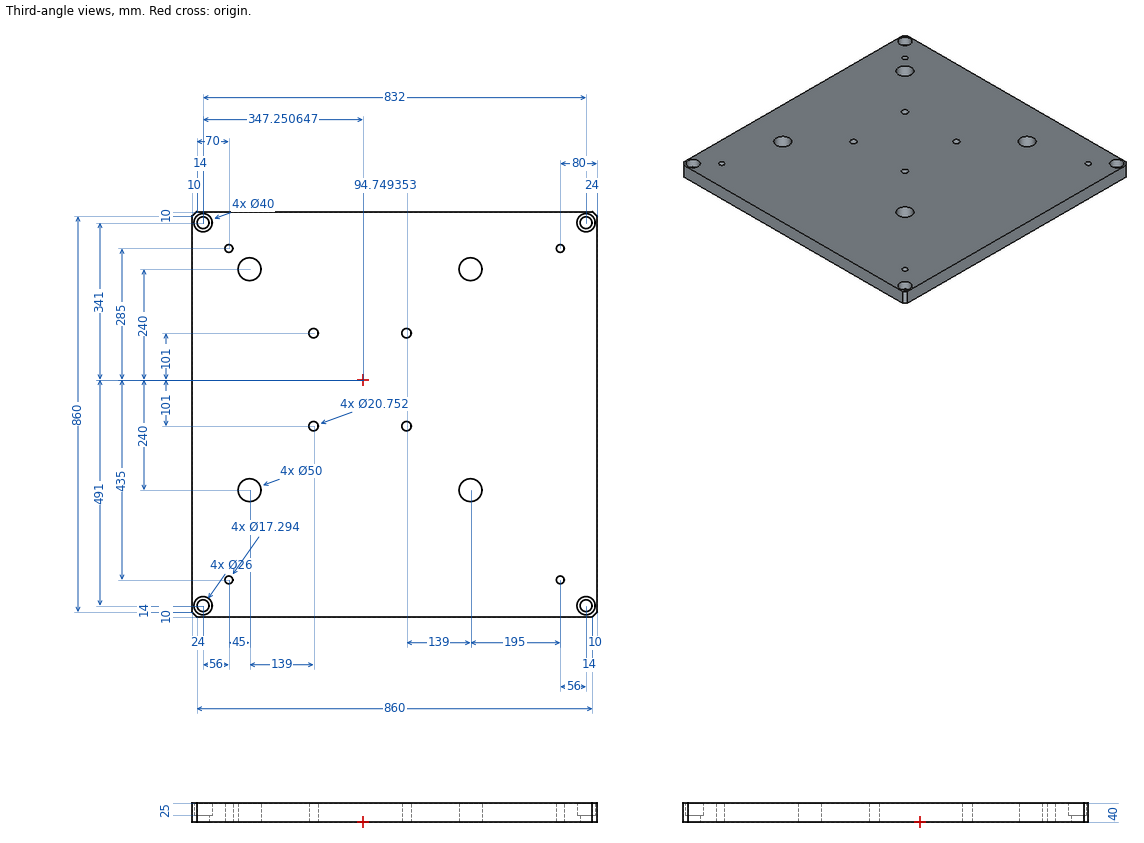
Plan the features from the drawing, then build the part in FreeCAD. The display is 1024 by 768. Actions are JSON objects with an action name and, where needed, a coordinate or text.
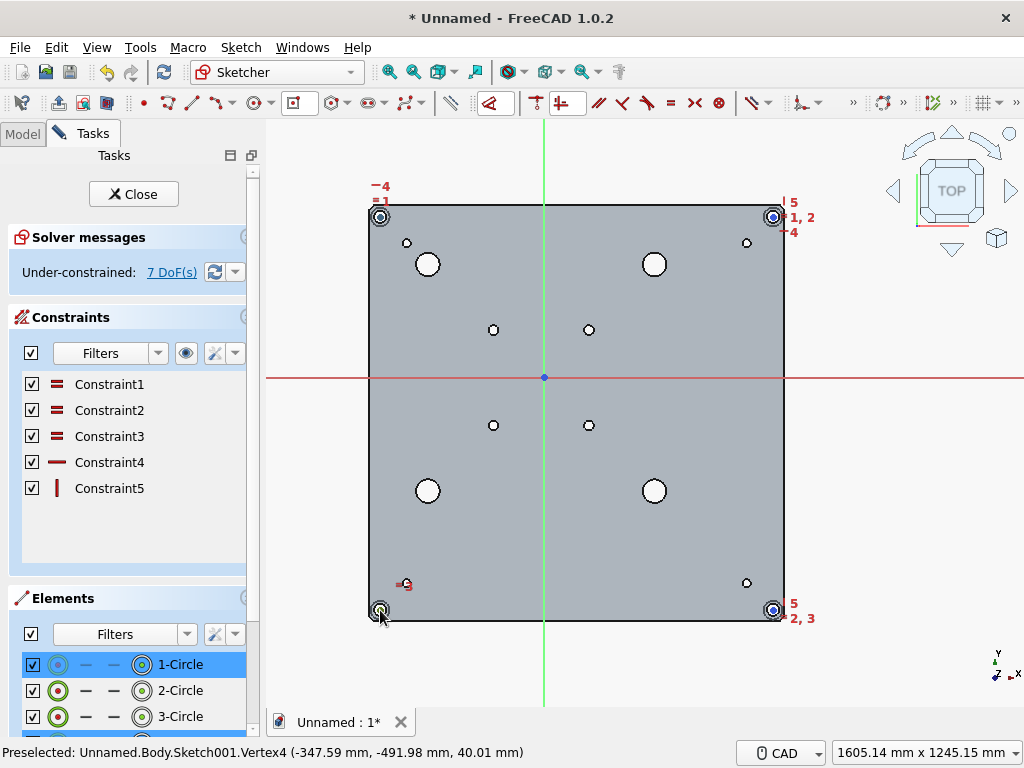
{"action": "key", "text": "v"}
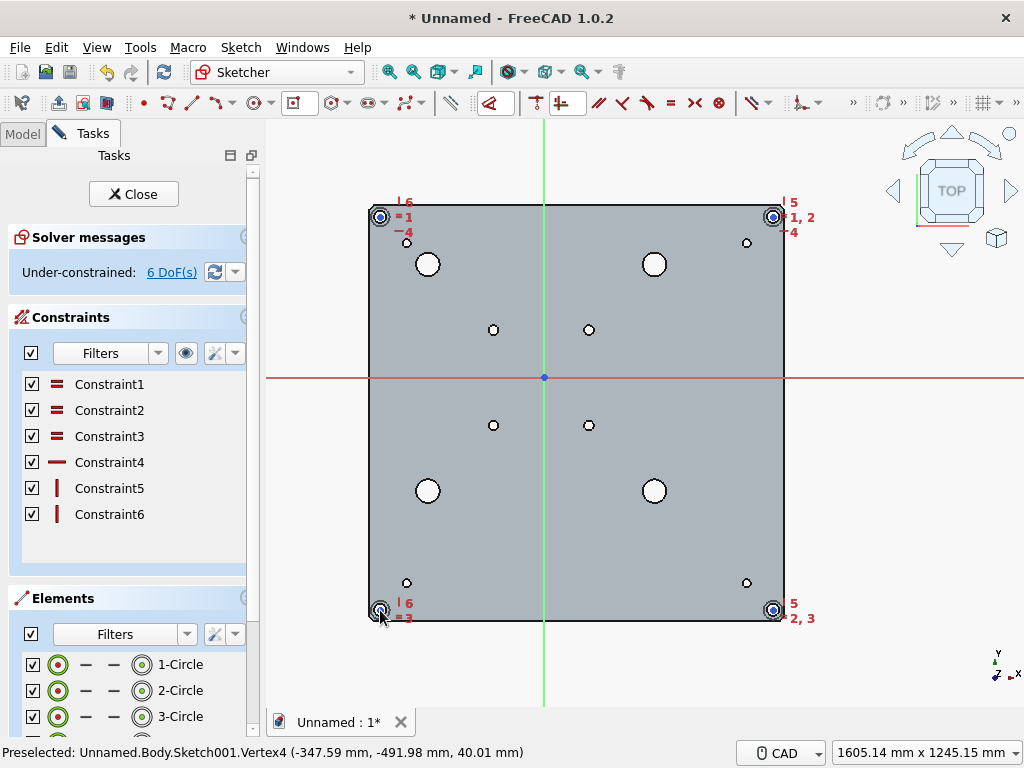
{"action": "left_click", "coordinate": [773, 610]}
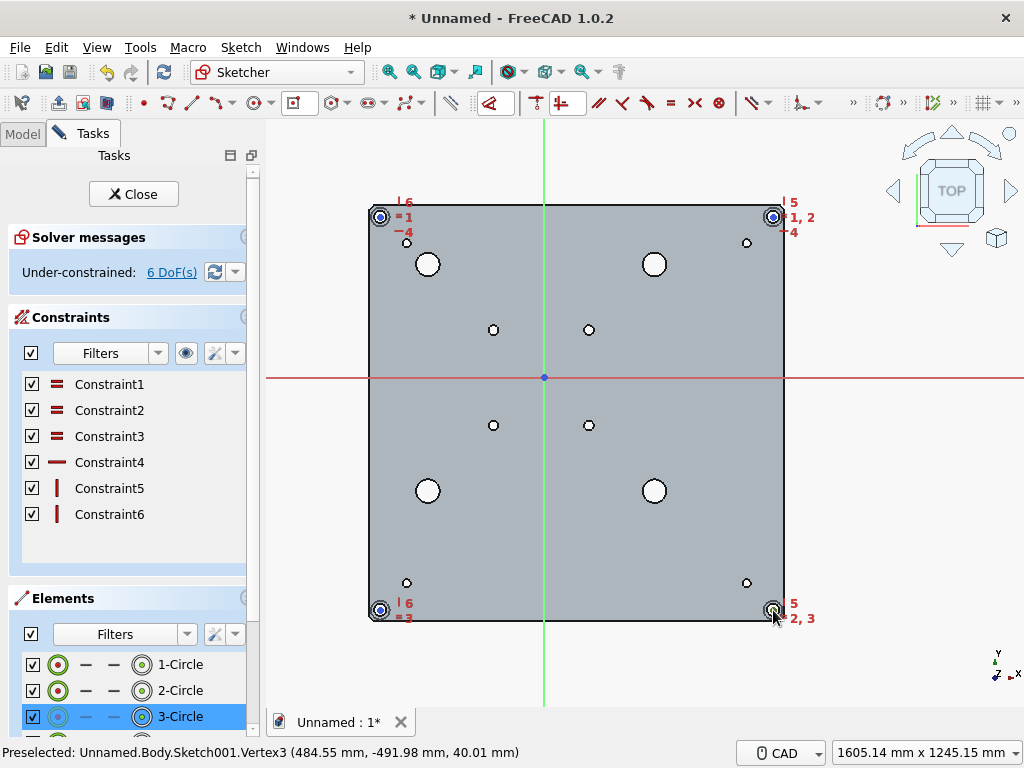
{"action": "left_click", "coordinate": [380, 610]}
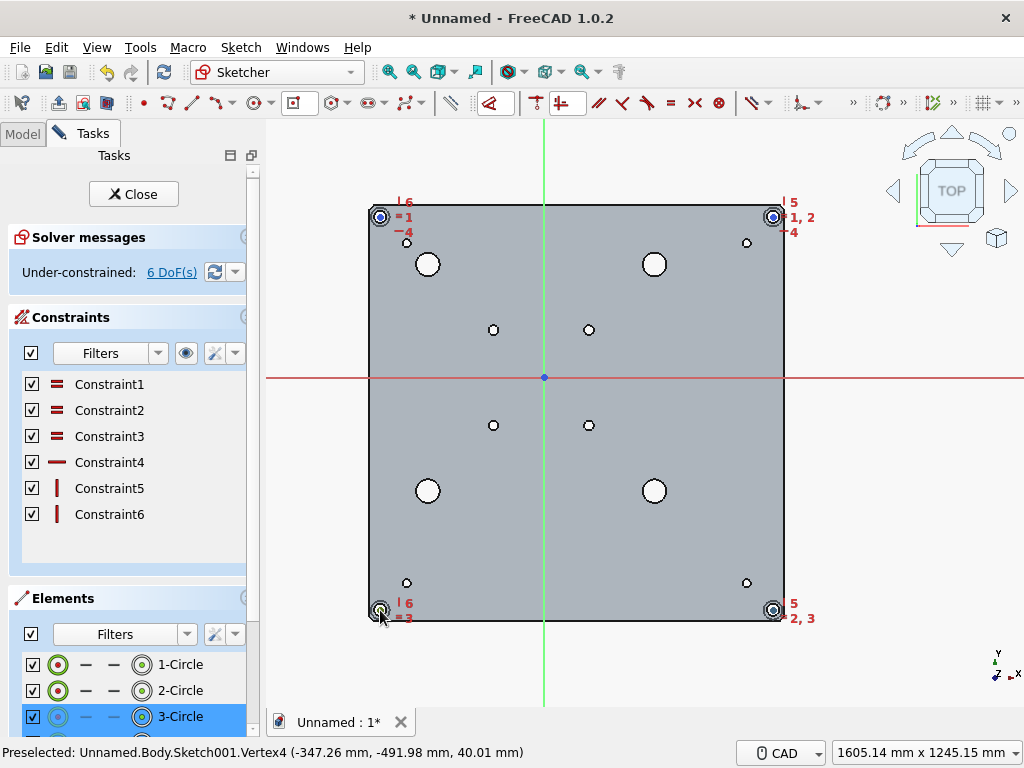
{"action": "key", "text": "h"}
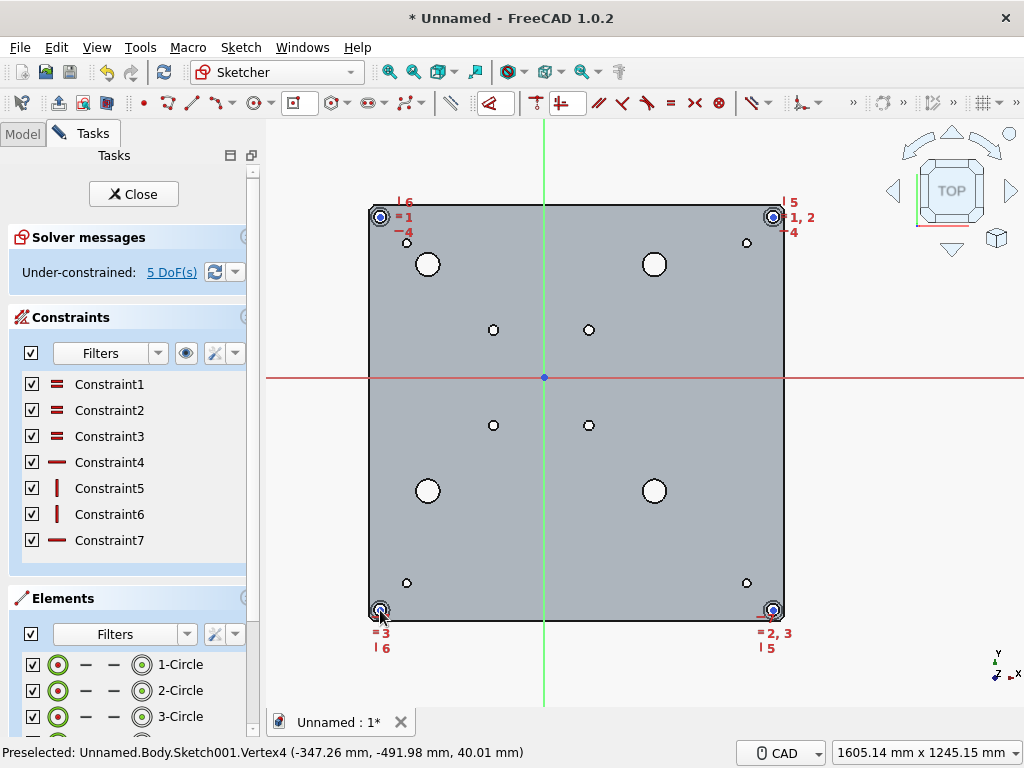
{"action": "scroll", "coordinate": [387, 210], "scroll_direction": "up", "scroll_amount": 4}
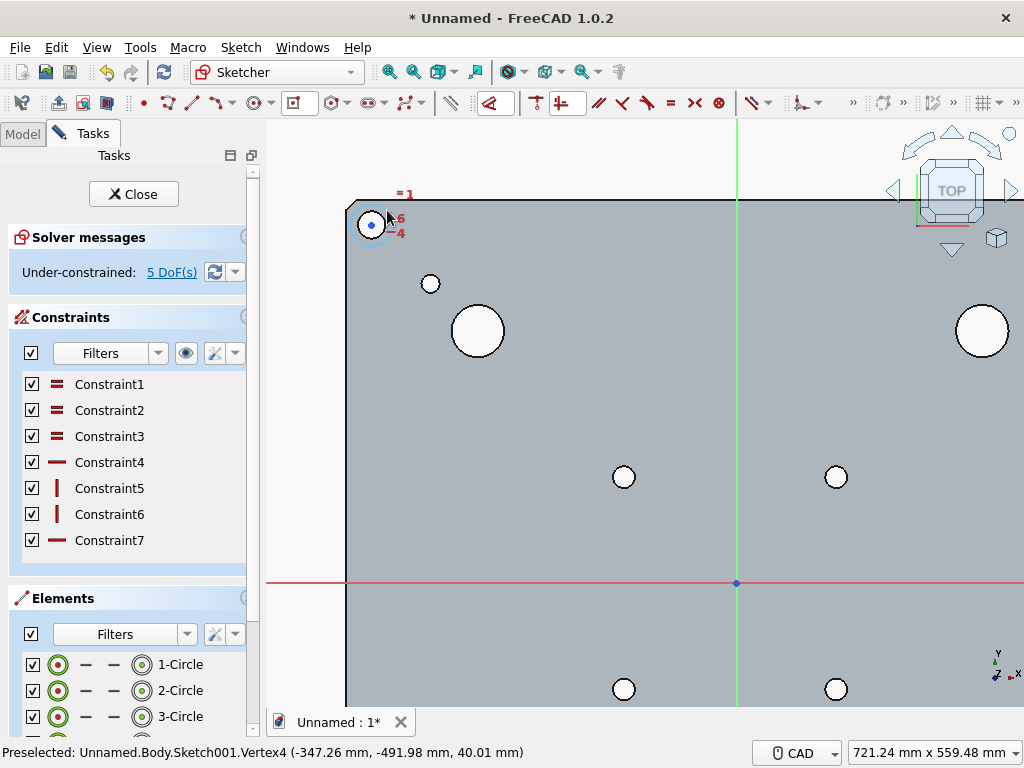
{"action": "left_click", "coordinate": [357, 211]}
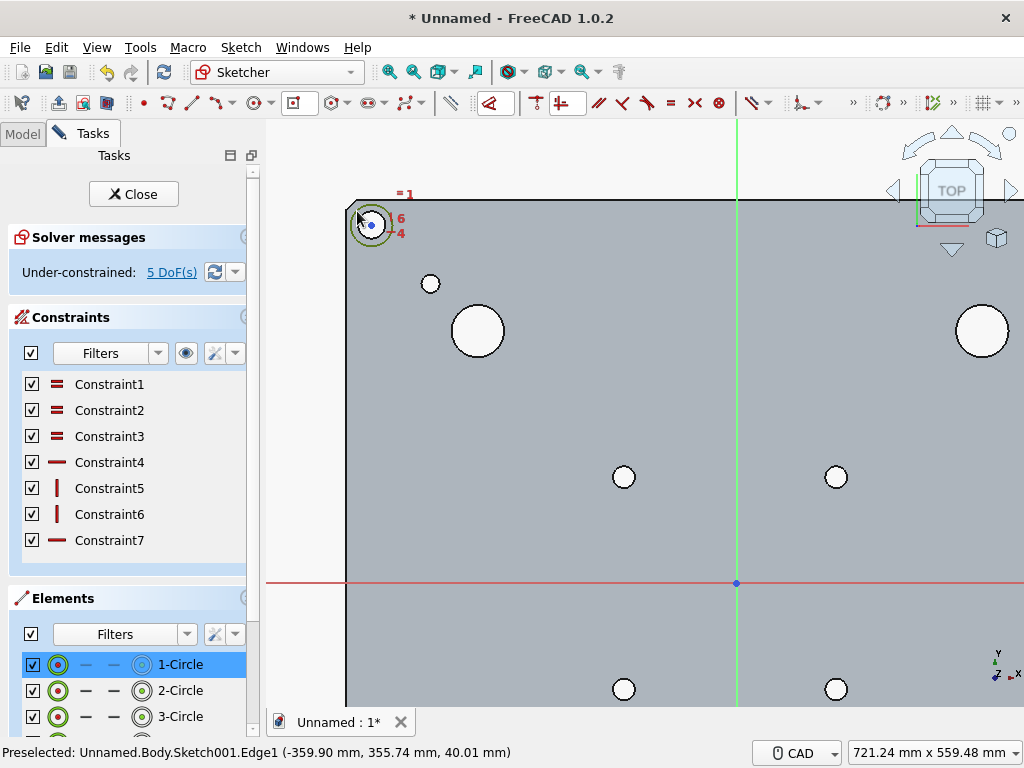
{"action": "left_click", "coordinate": [508, 104]}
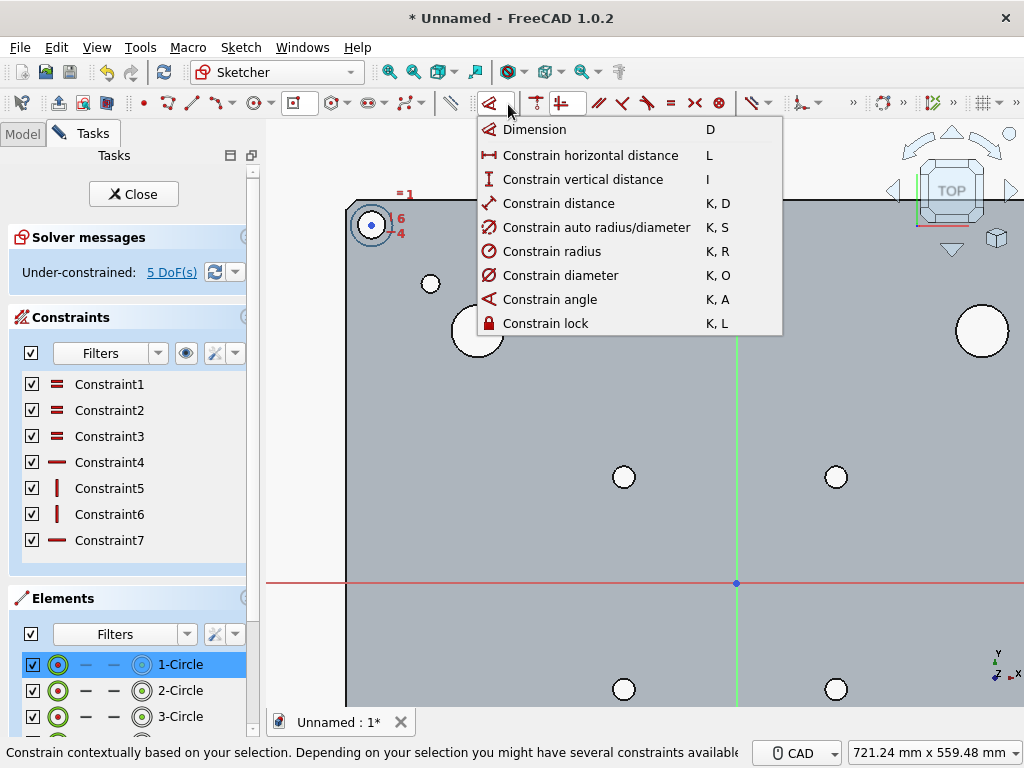
{"action": "left_click", "coordinate": [630, 275]}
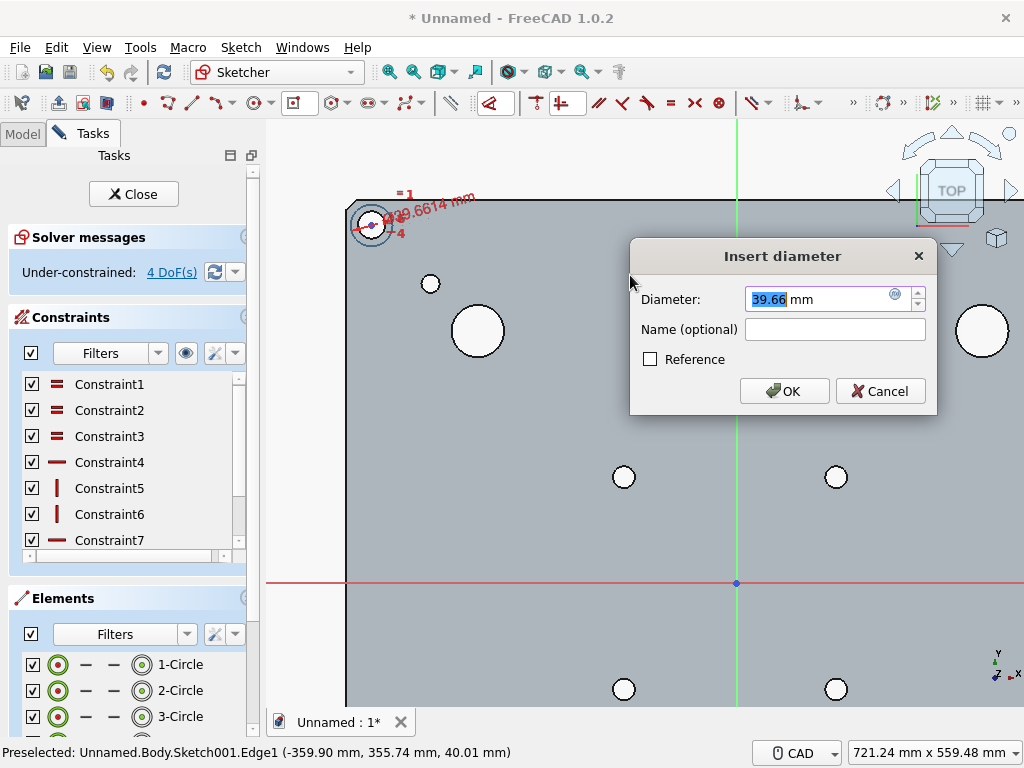
{"action": "type", "text": "40"}
{"action": "key", "text": "Return"}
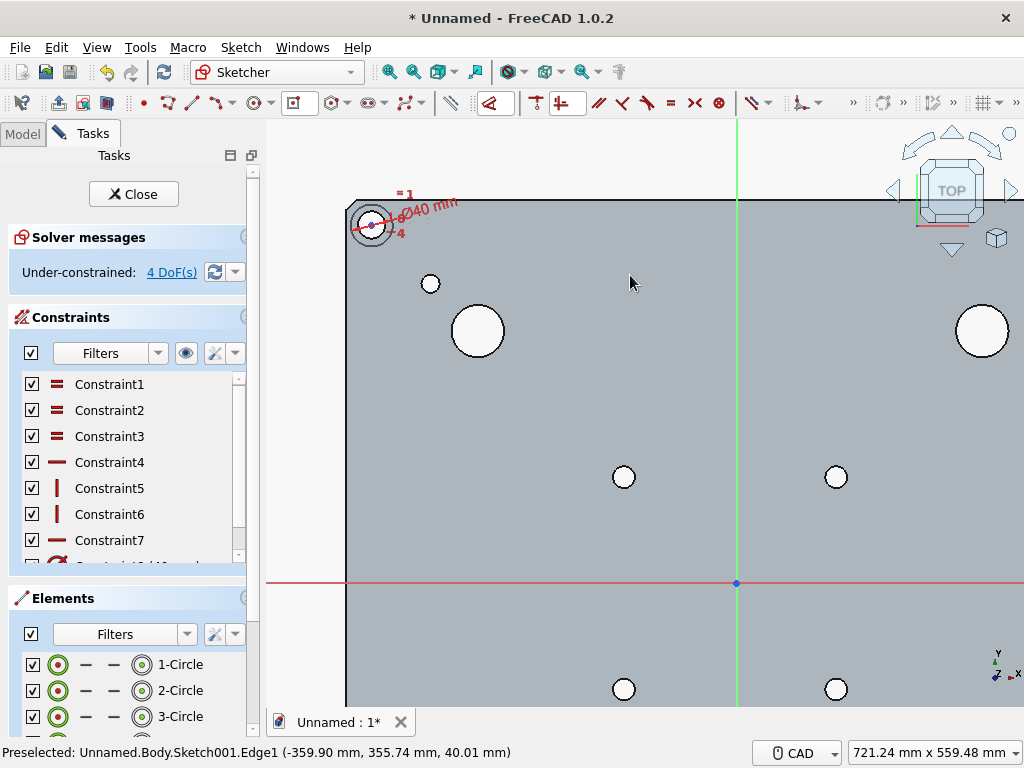
{"action": "left_click", "coordinate": [372, 226]}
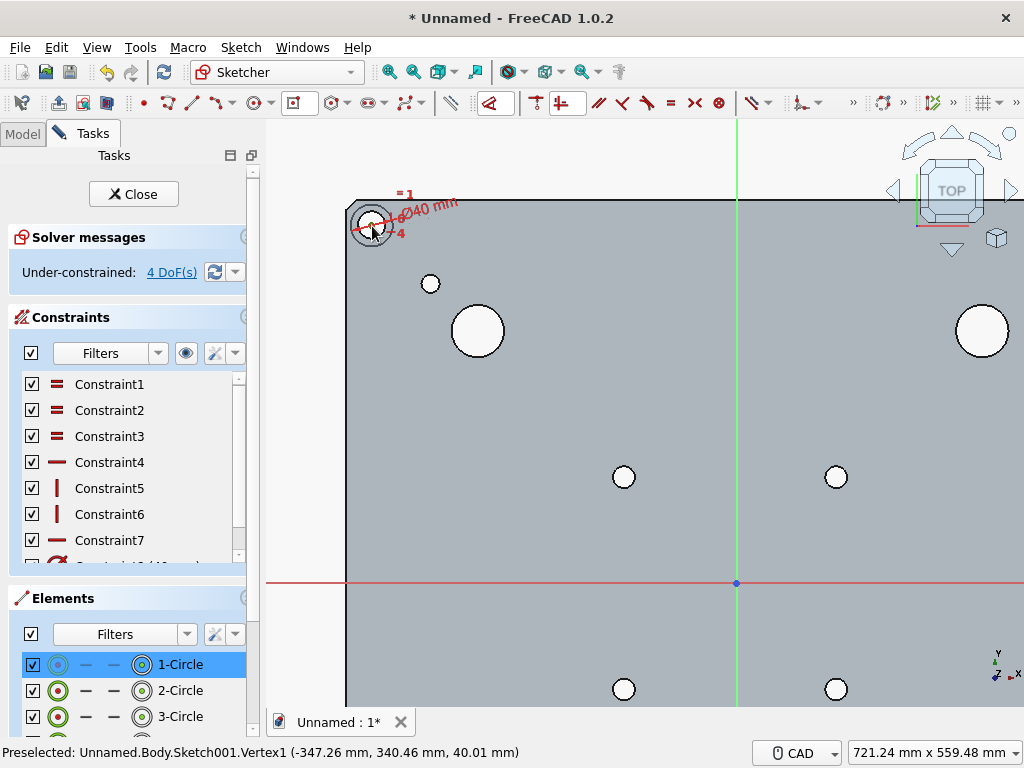
{"action": "key", "text": "i"}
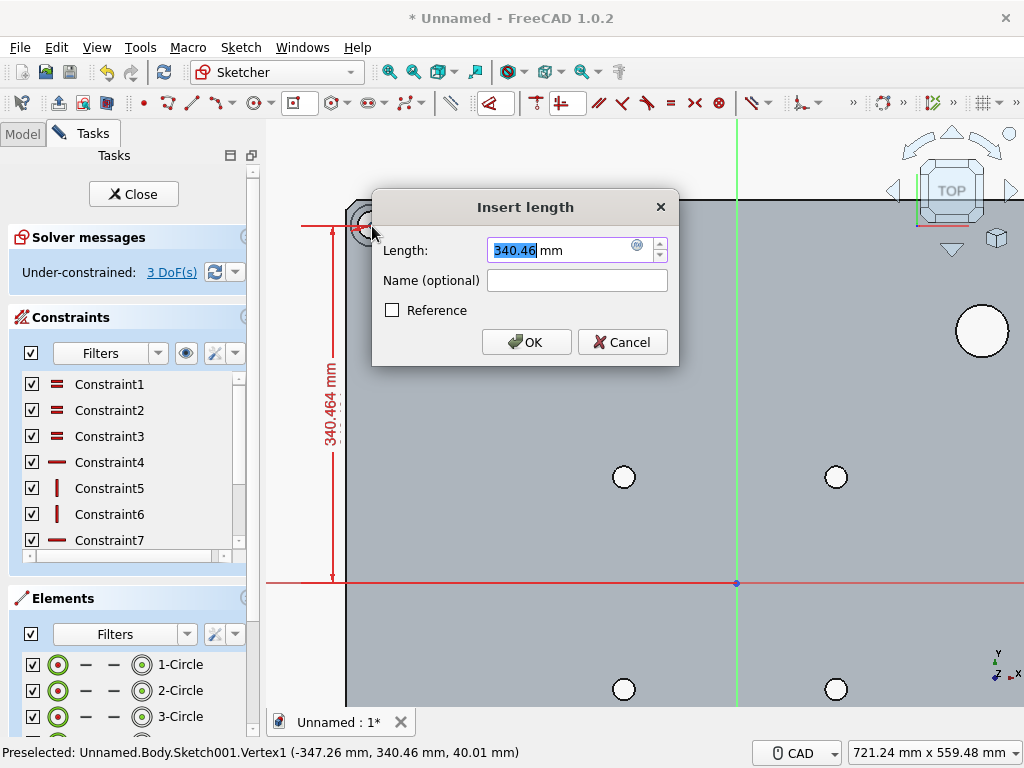
{"action": "type", "text": "341"}
{"action": "key", "text": "Return"}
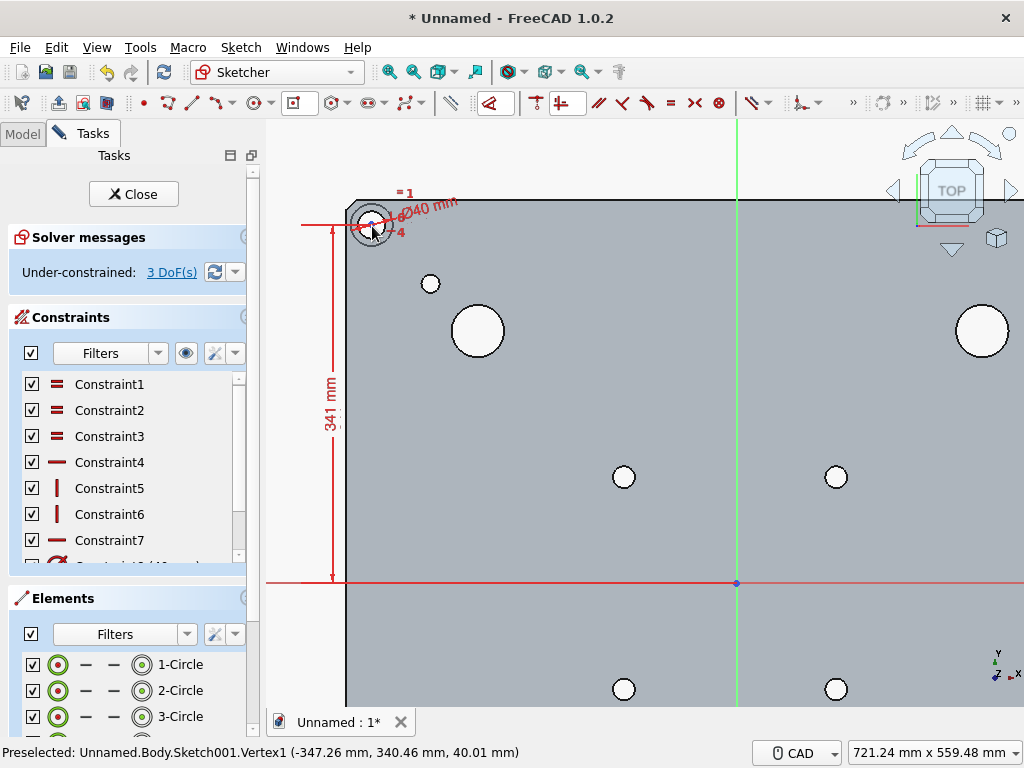
{"action": "scroll", "coordinate": [387, 210], "scroll_direction": "down", "scroll_amount": 4}